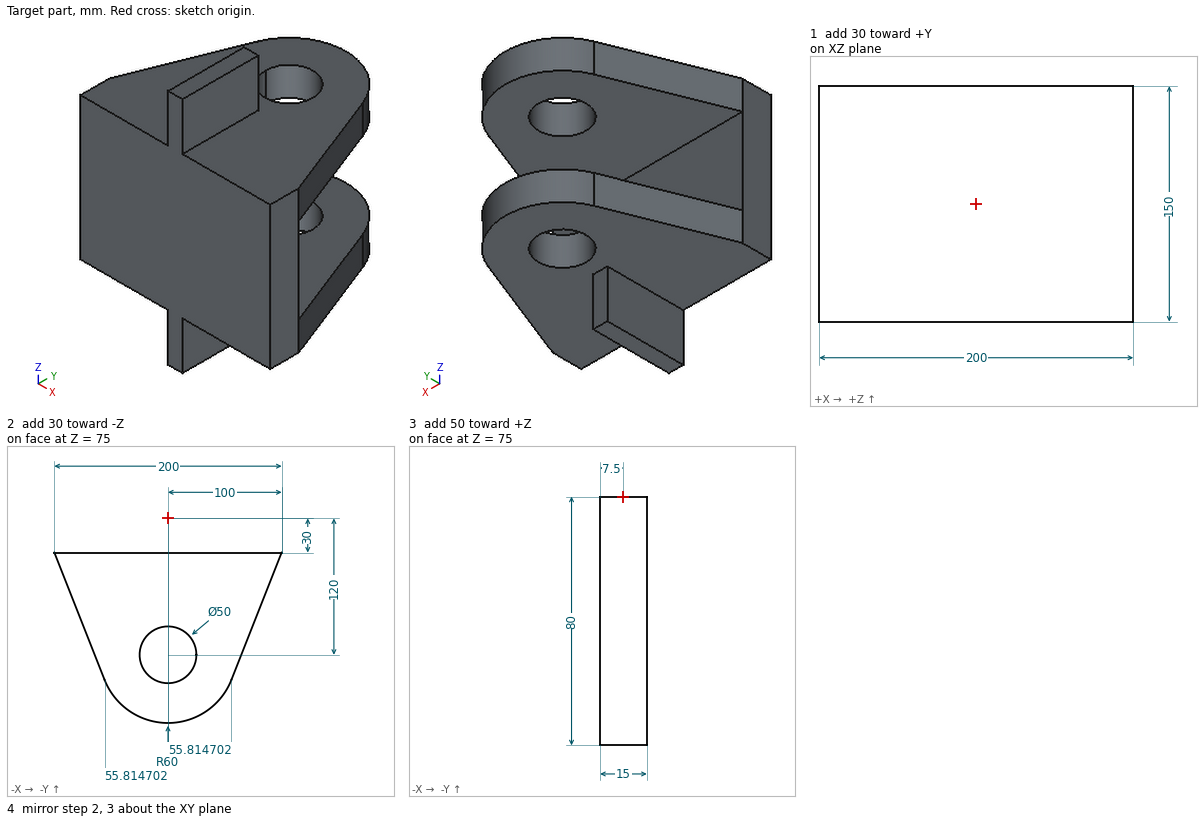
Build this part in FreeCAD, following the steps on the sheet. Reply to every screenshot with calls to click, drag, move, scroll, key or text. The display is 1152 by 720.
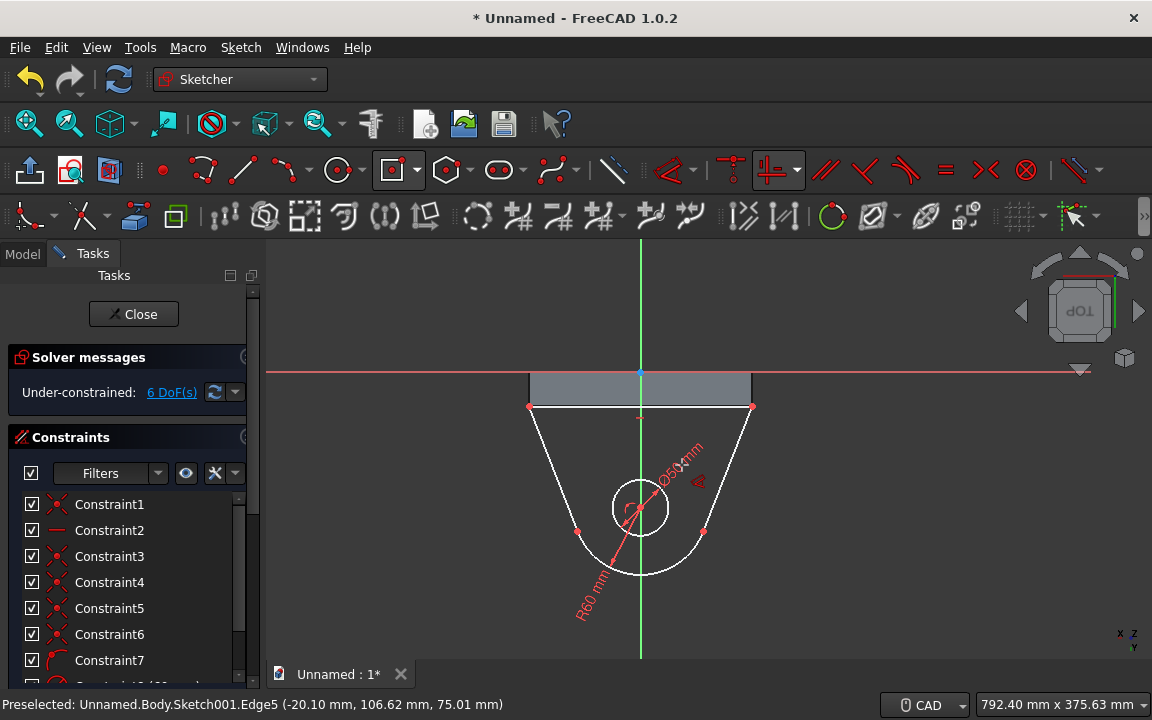
click(685, 407)
click(589, 441)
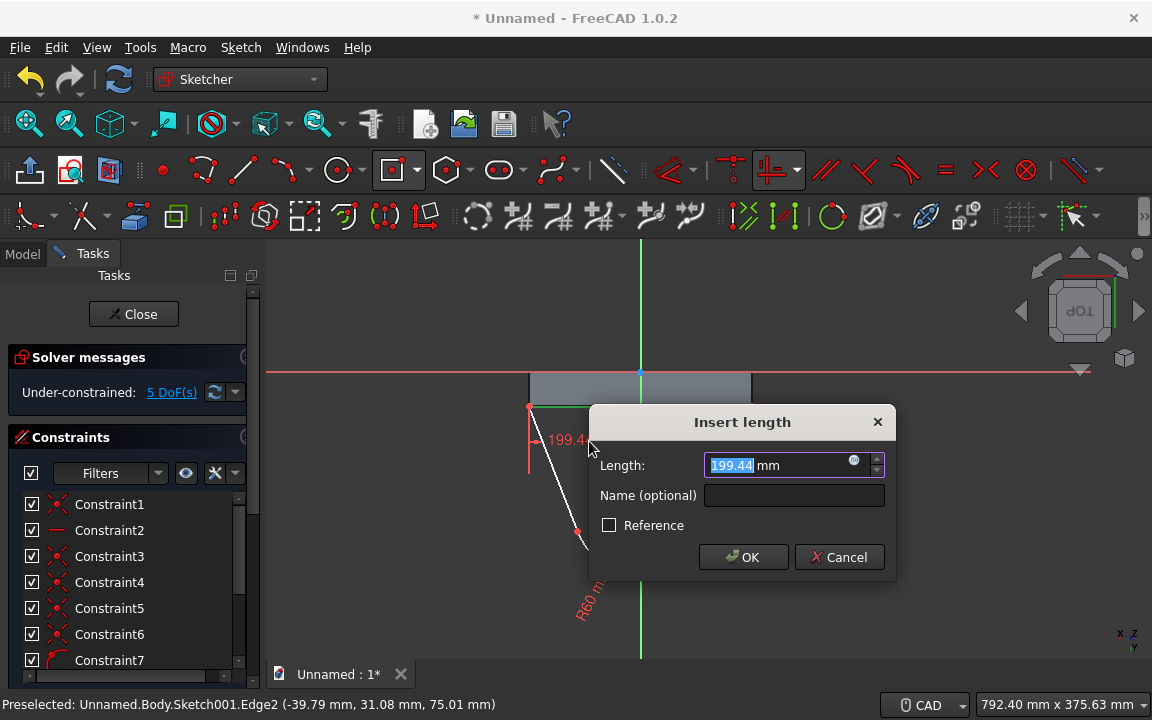
text(200)
key(Return)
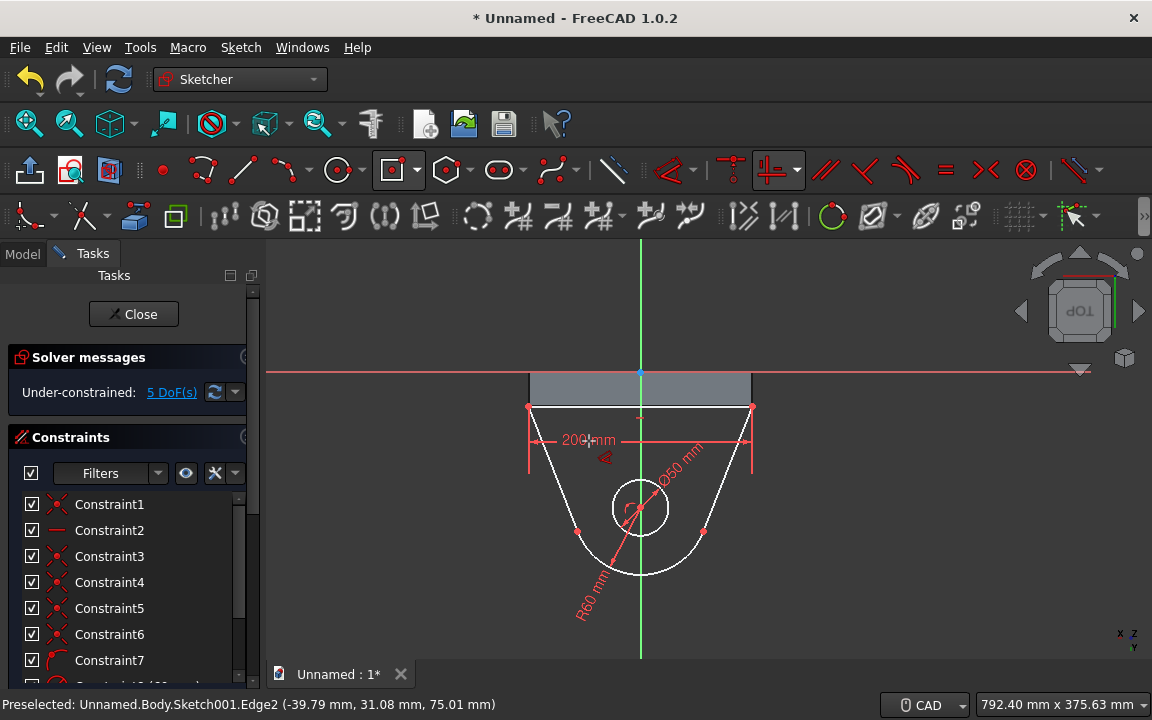
click(752, 407)
click(786, 390)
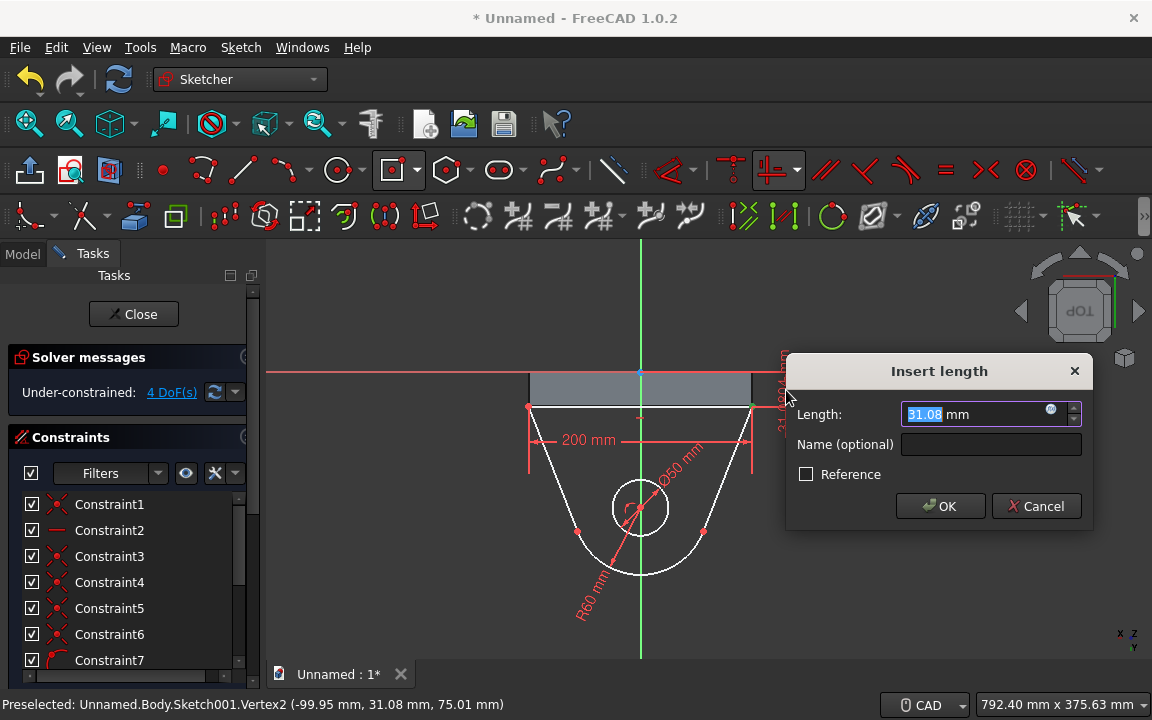
text(30)
key(Return)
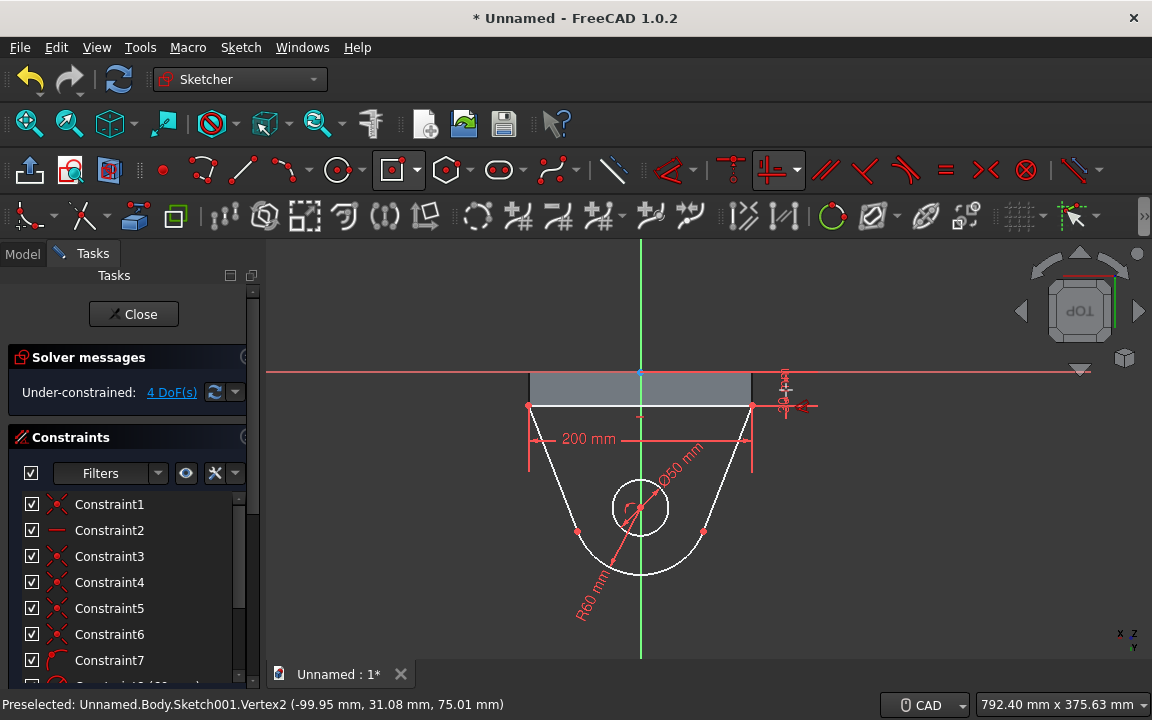
click(641, 508)
click(675, 440)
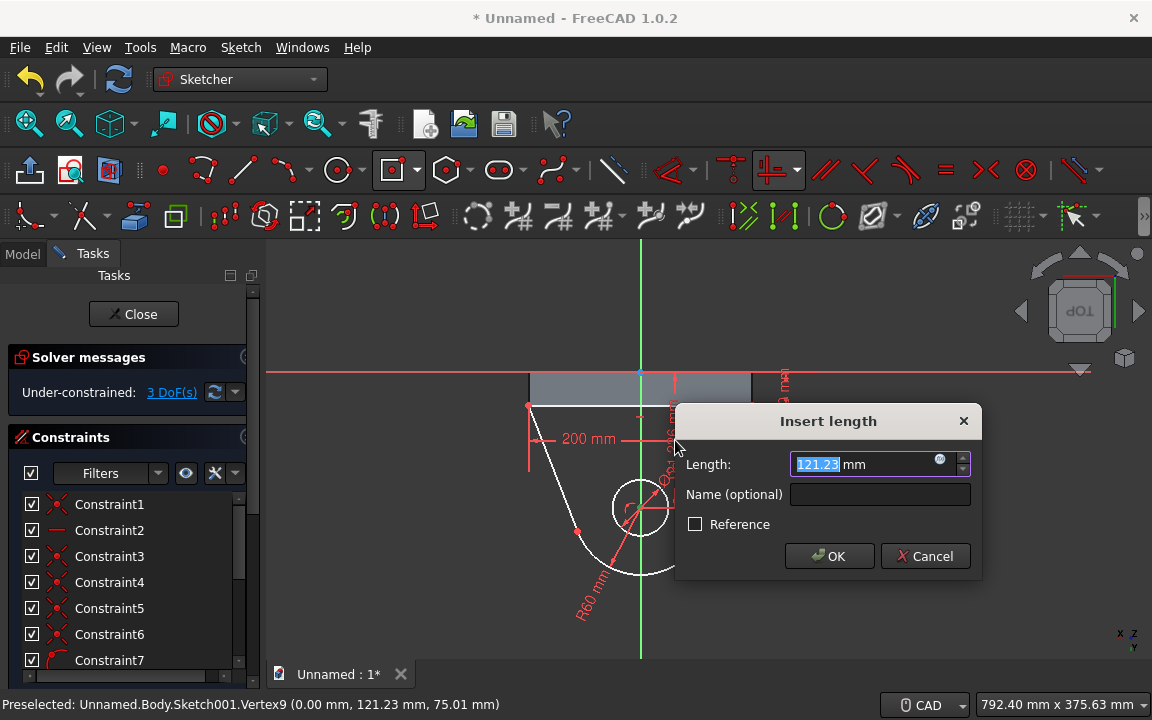
text(120)
key(Return)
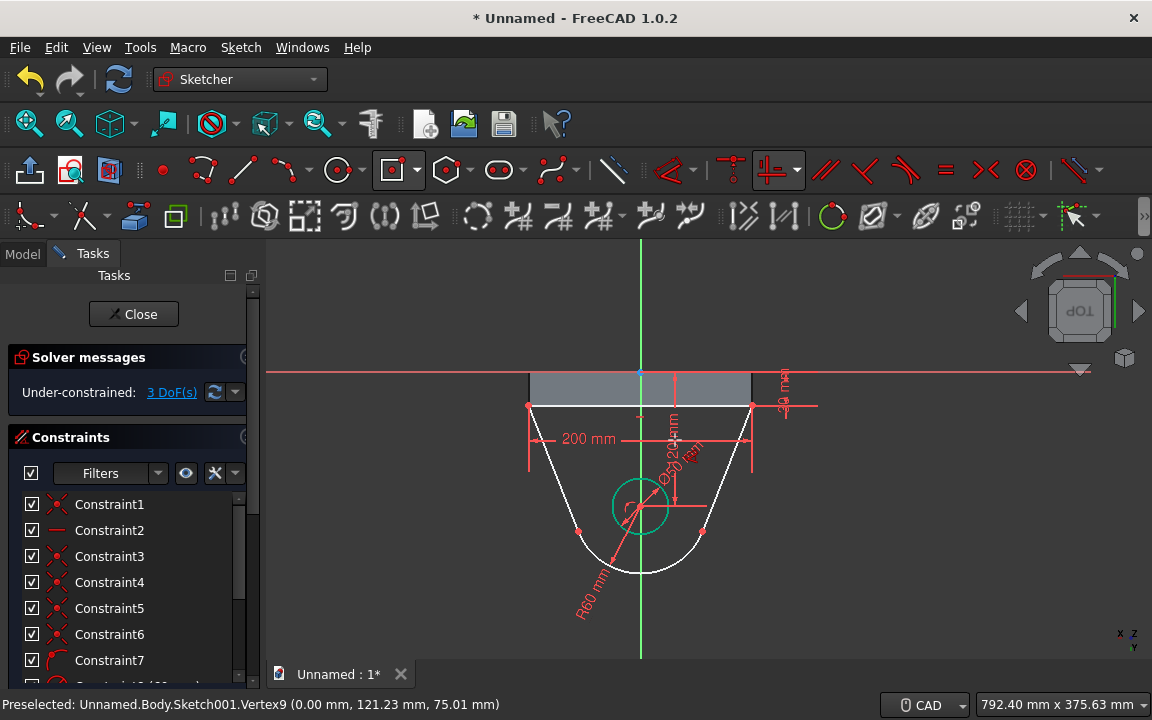
click(752, 406)
click(696, 338)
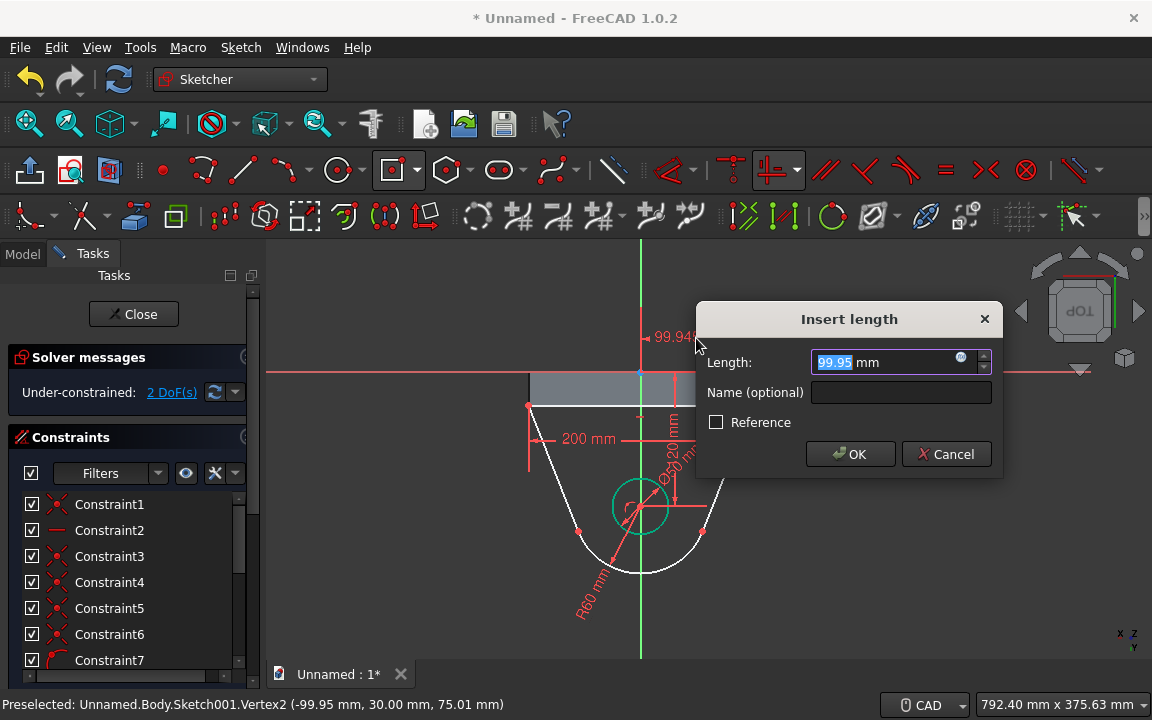
text(100)
key(Return)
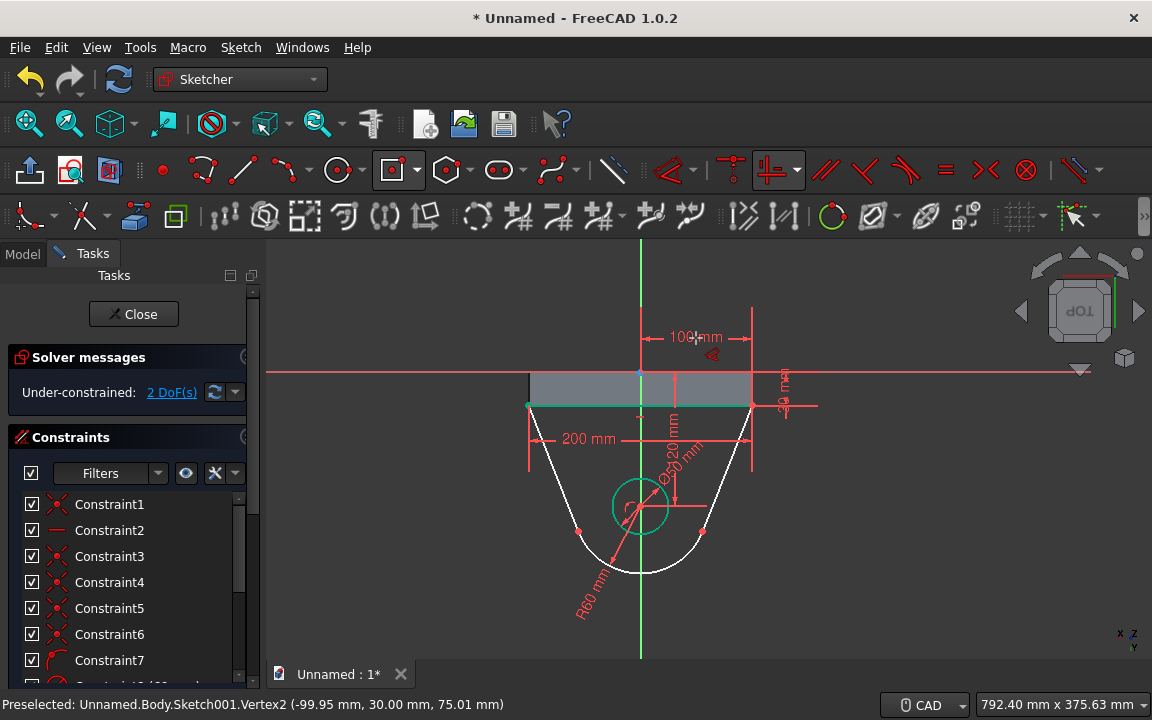
click(703, 532)
click(672, 314)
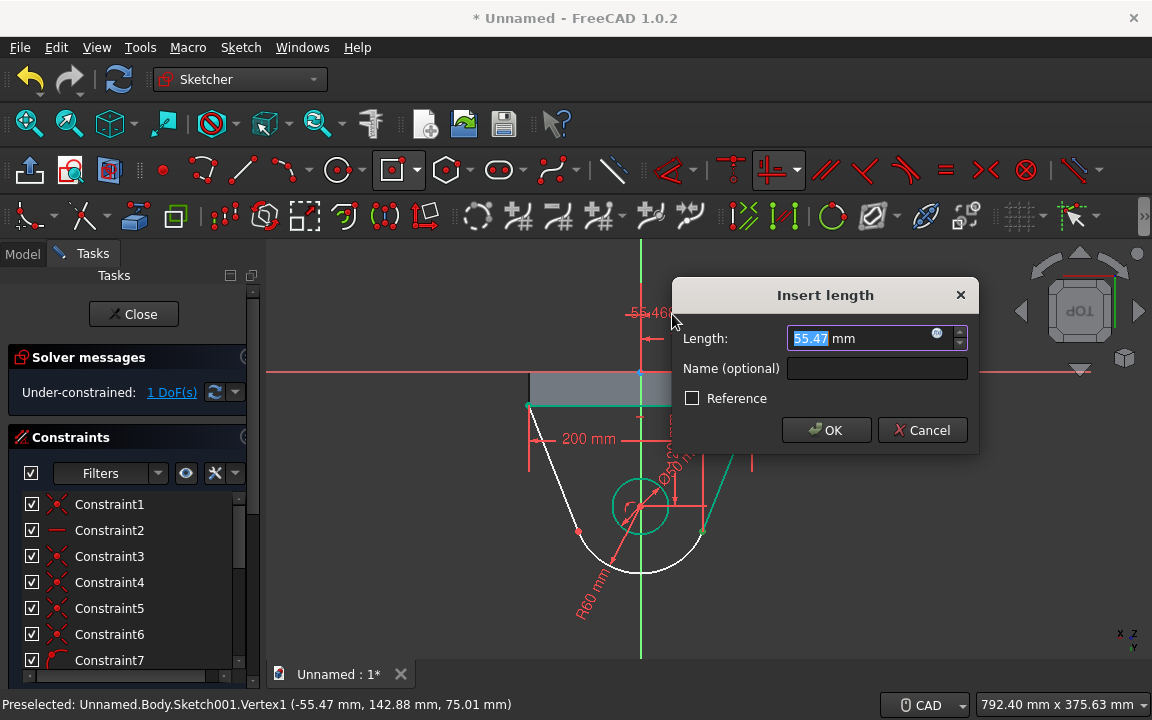
text(55.814702)
key(Return)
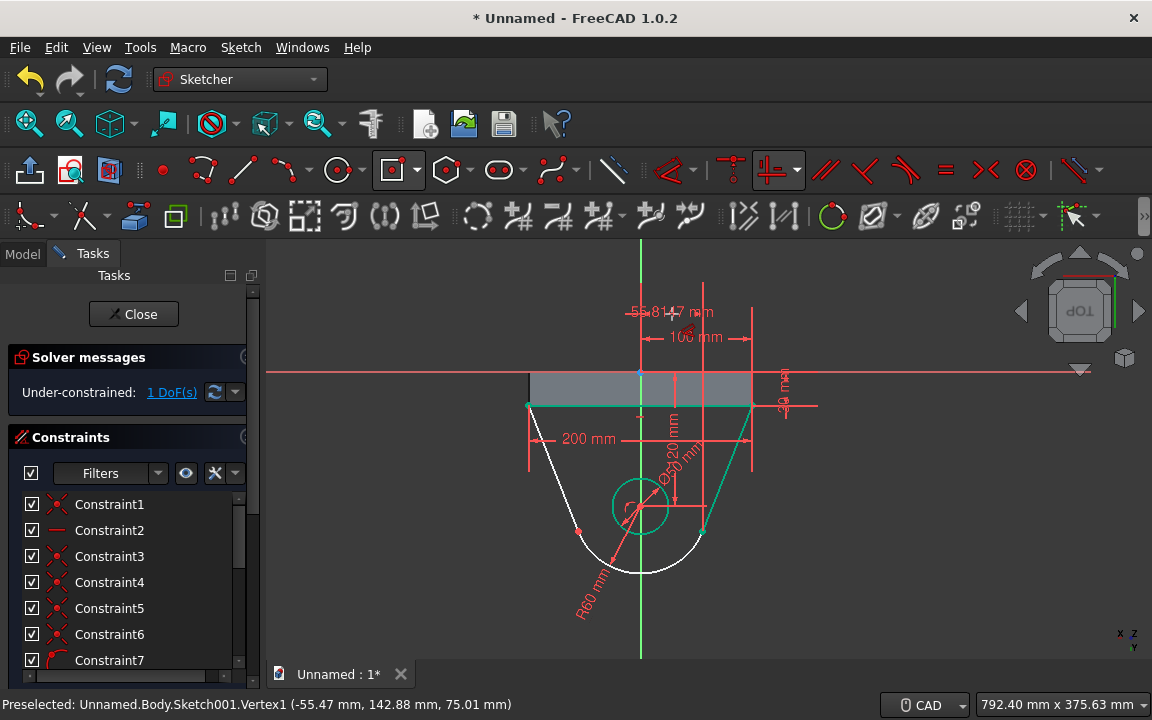
click(578, 532)
click(610, 338)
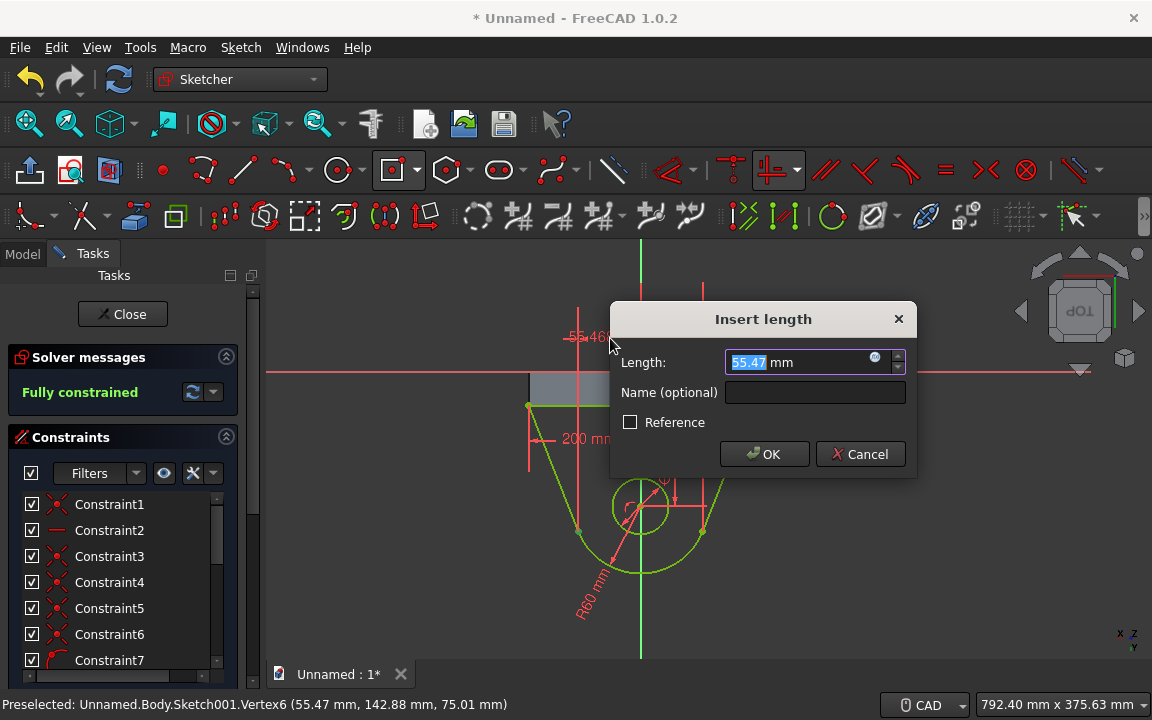
text(55.814702)
key(Return)
key(Escape)